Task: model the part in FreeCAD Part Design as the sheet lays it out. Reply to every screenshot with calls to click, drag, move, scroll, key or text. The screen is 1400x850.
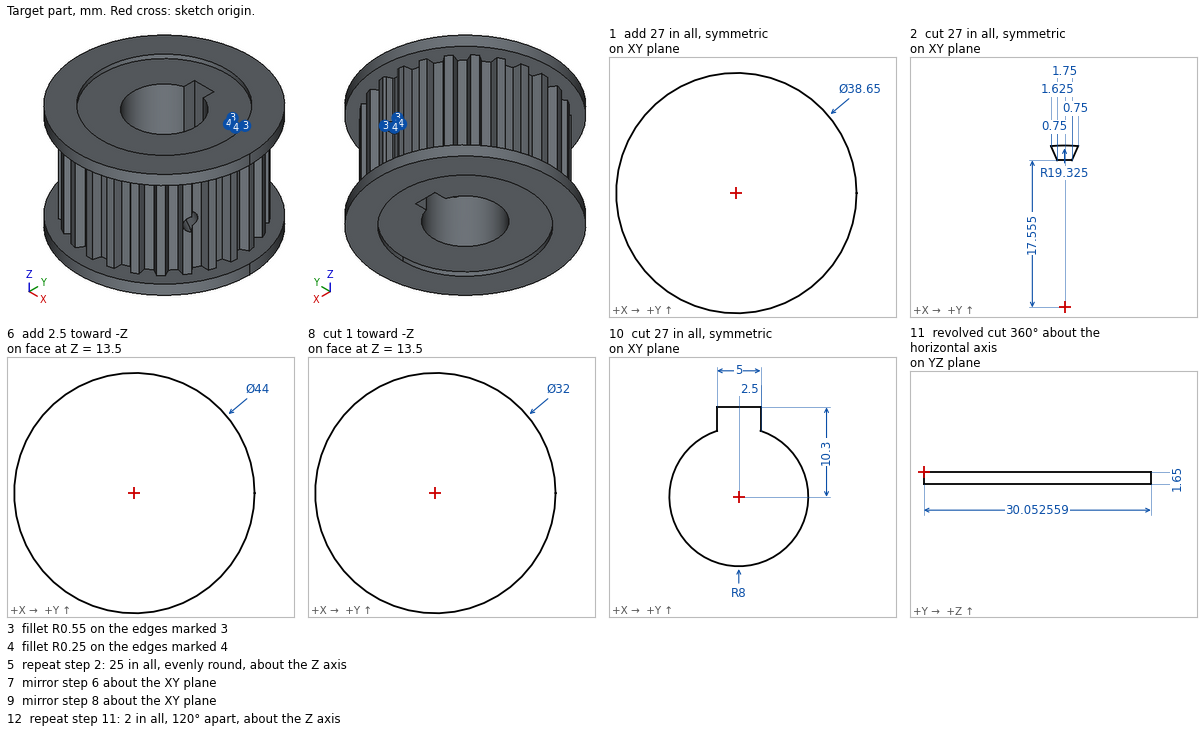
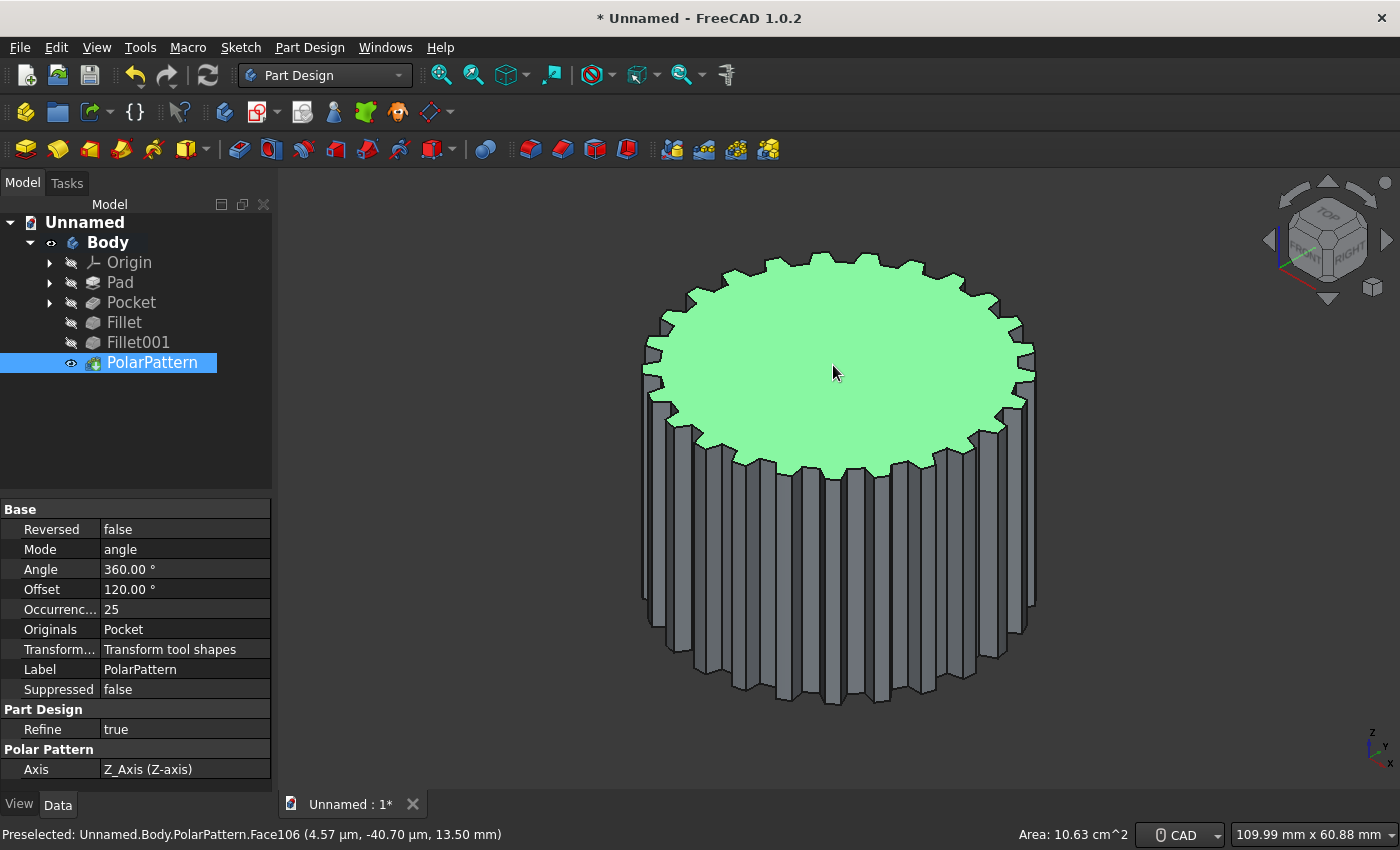
click(258, 112)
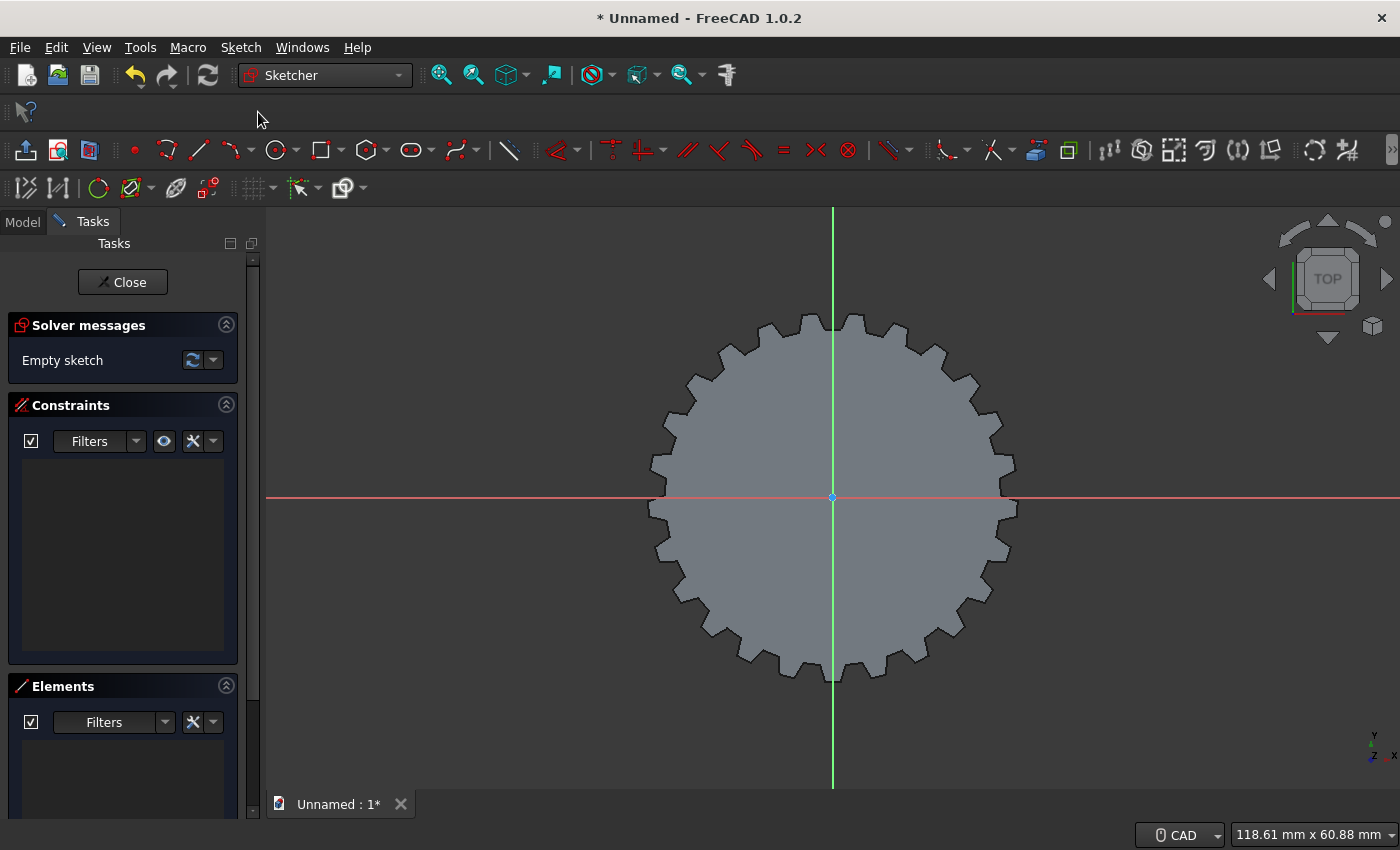
click(276, 150)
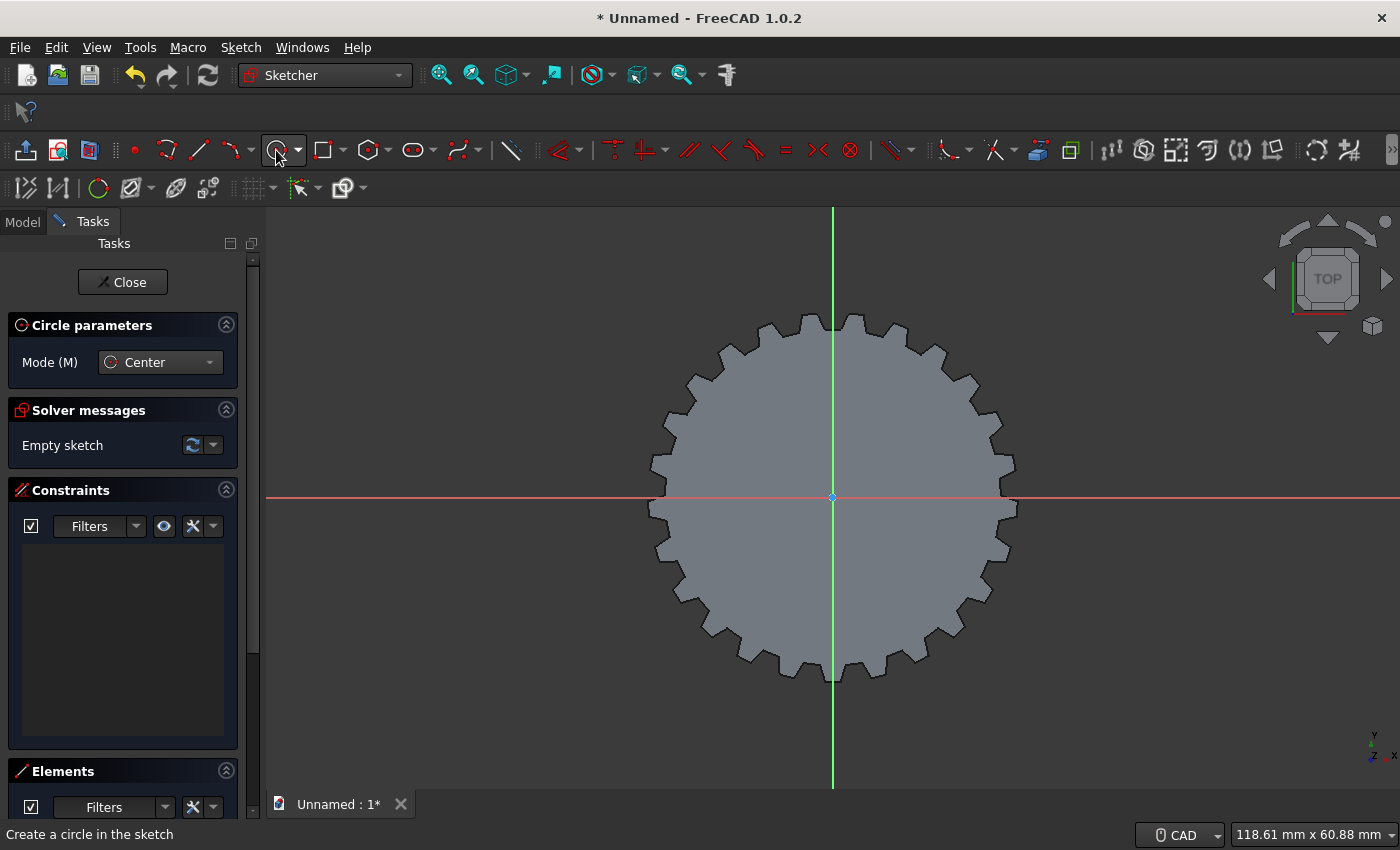
click(833, 498)
move(982, 349)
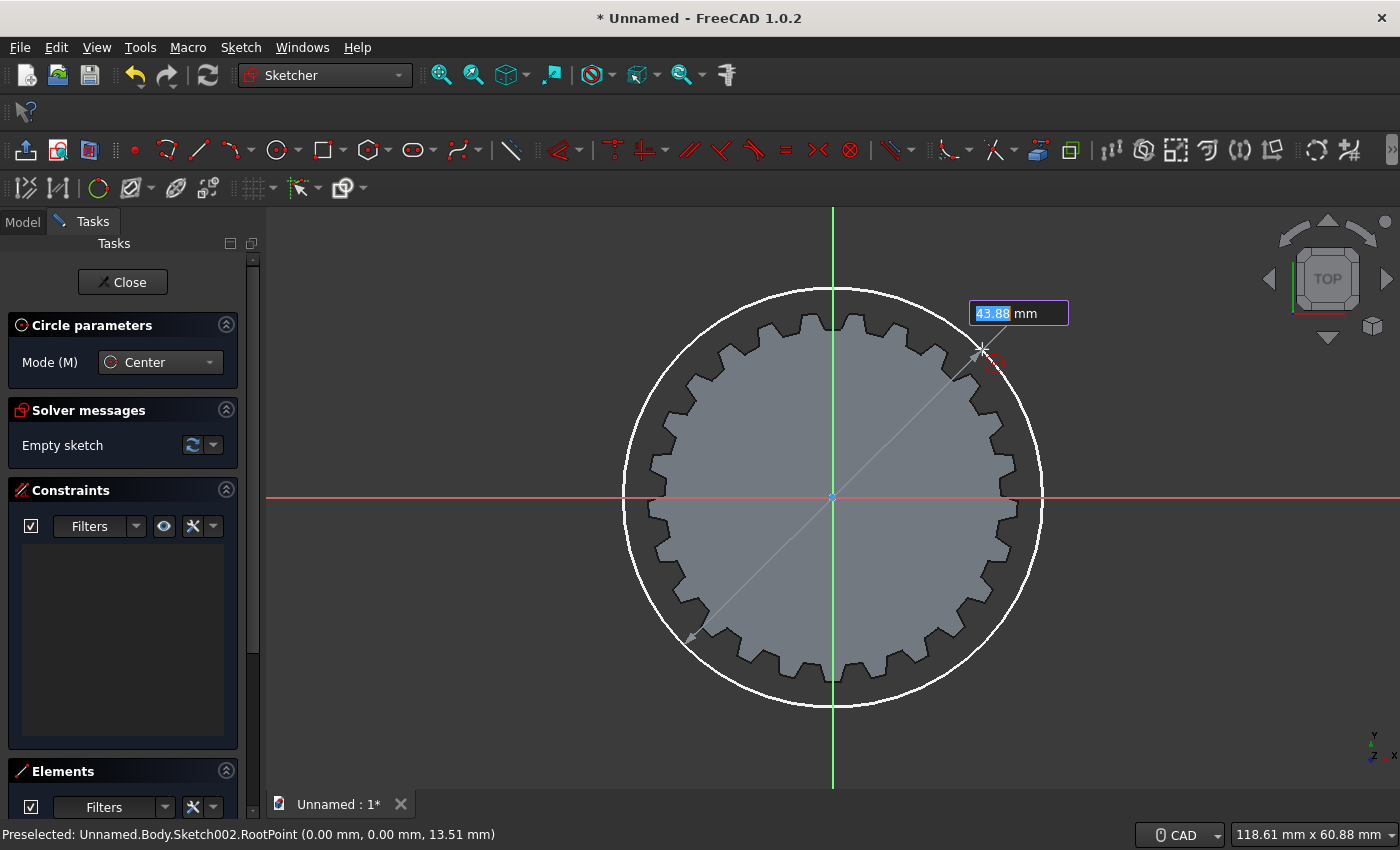
text(44)
key(Return)
key(Escape)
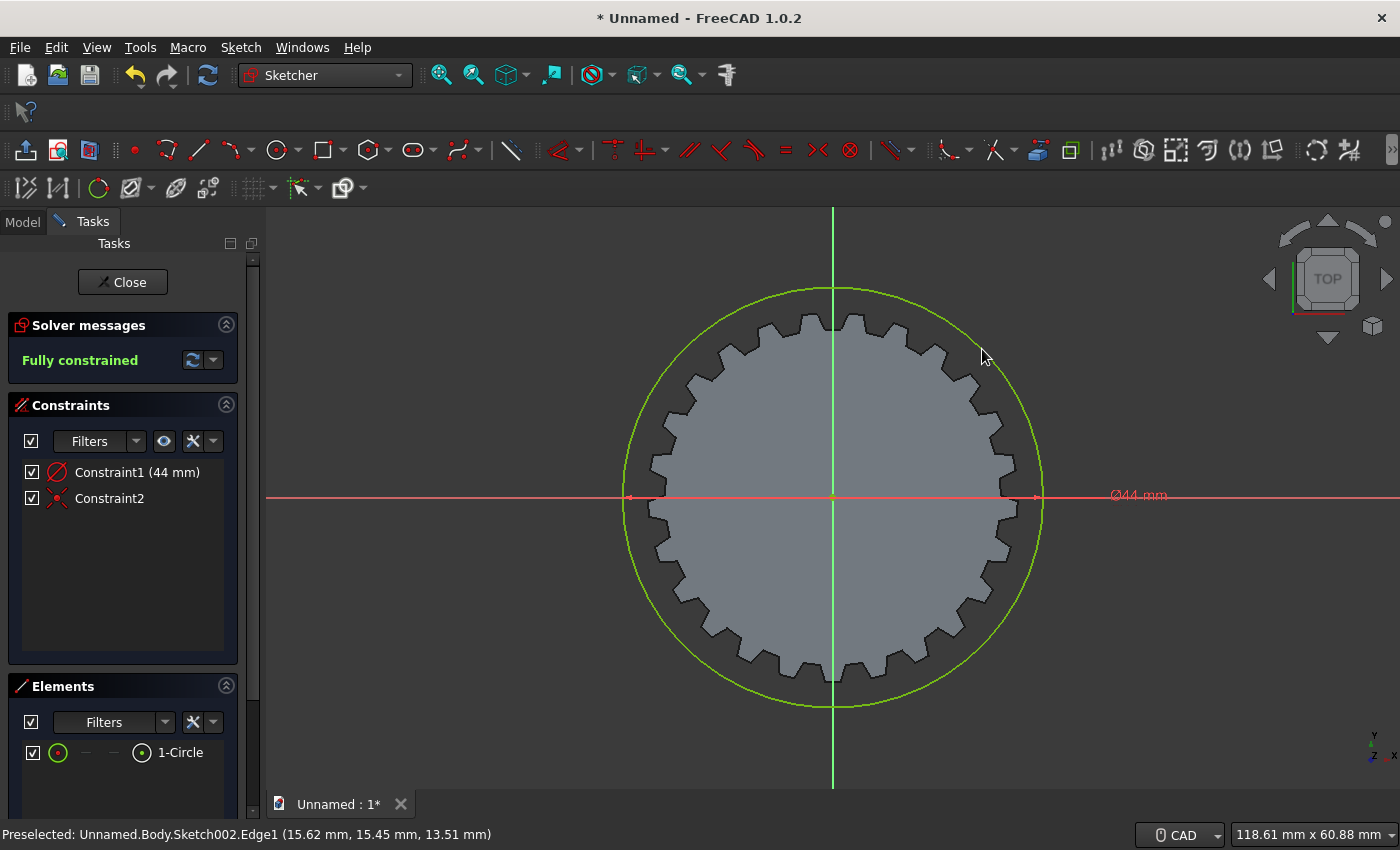
click(123, 282)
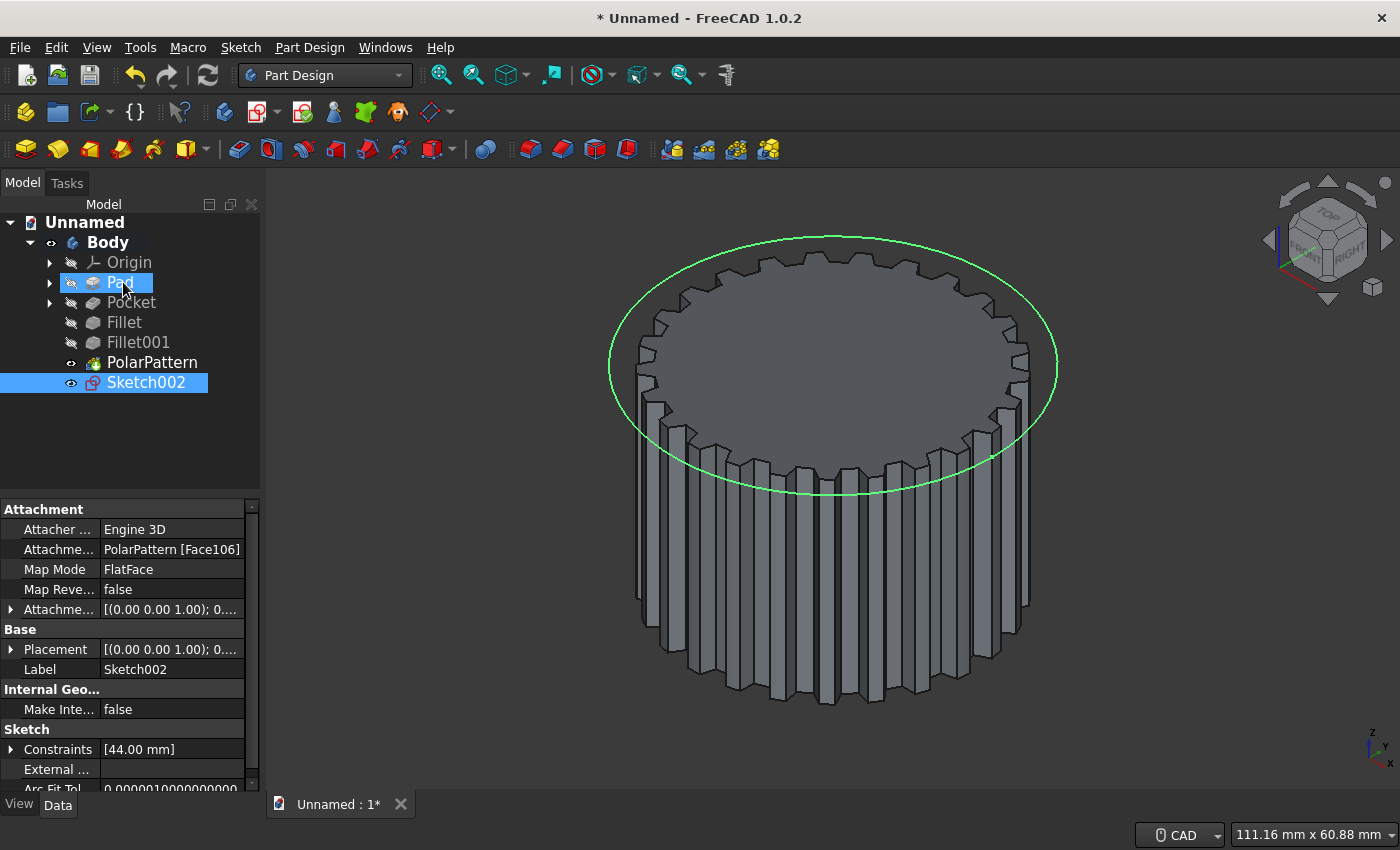
click(26, 150)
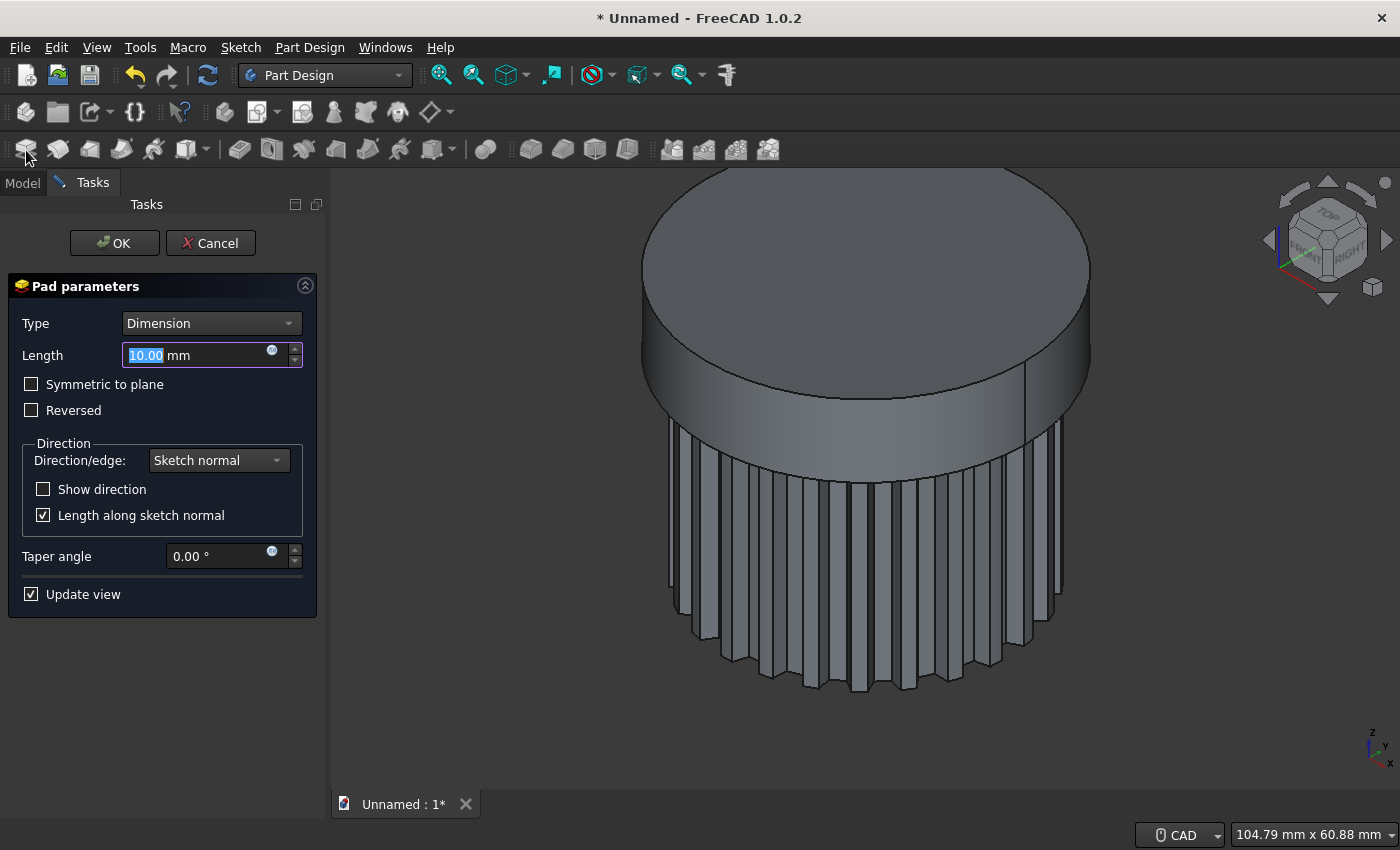
text(2.5)
key(Tab)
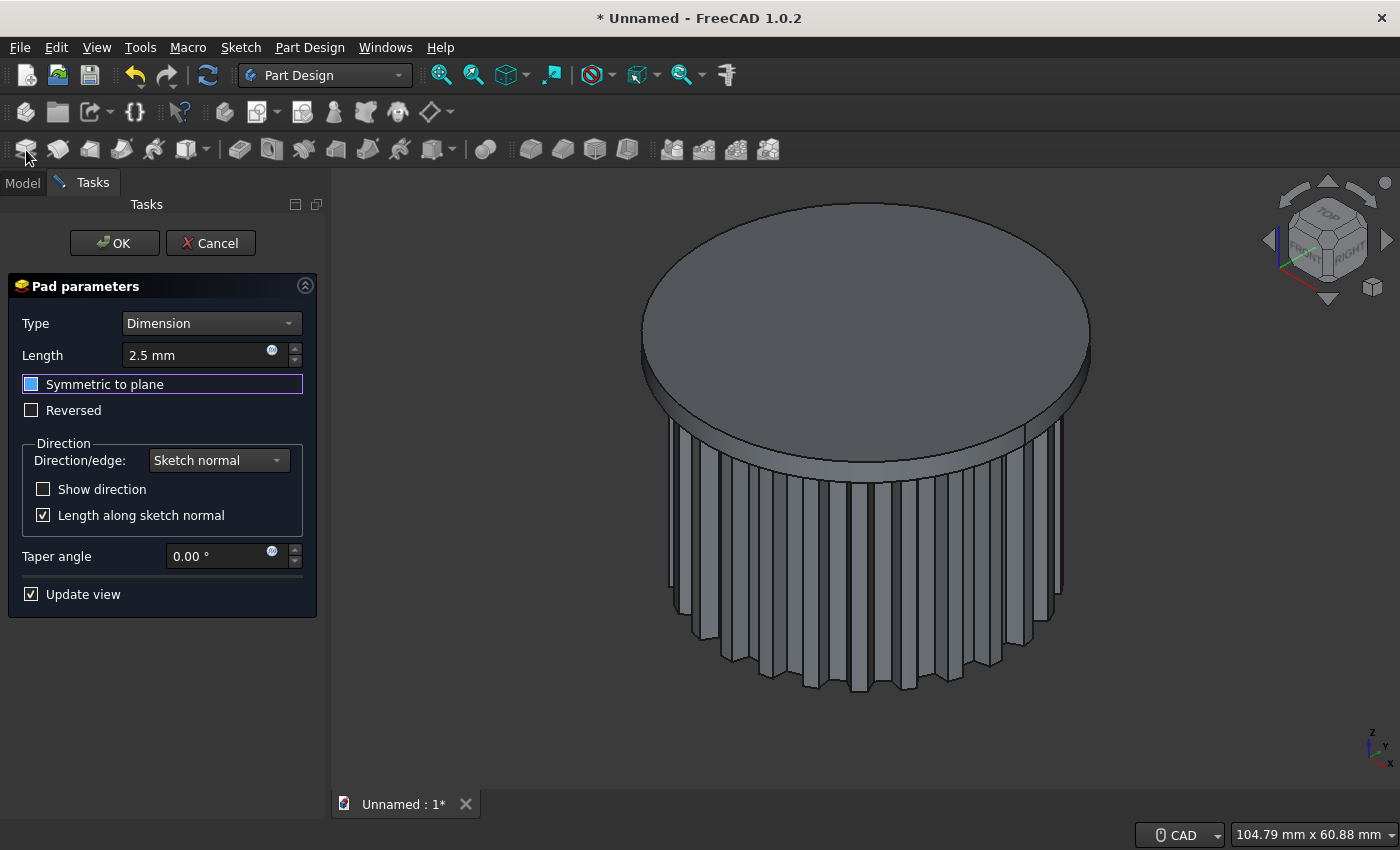
click(30, 410)